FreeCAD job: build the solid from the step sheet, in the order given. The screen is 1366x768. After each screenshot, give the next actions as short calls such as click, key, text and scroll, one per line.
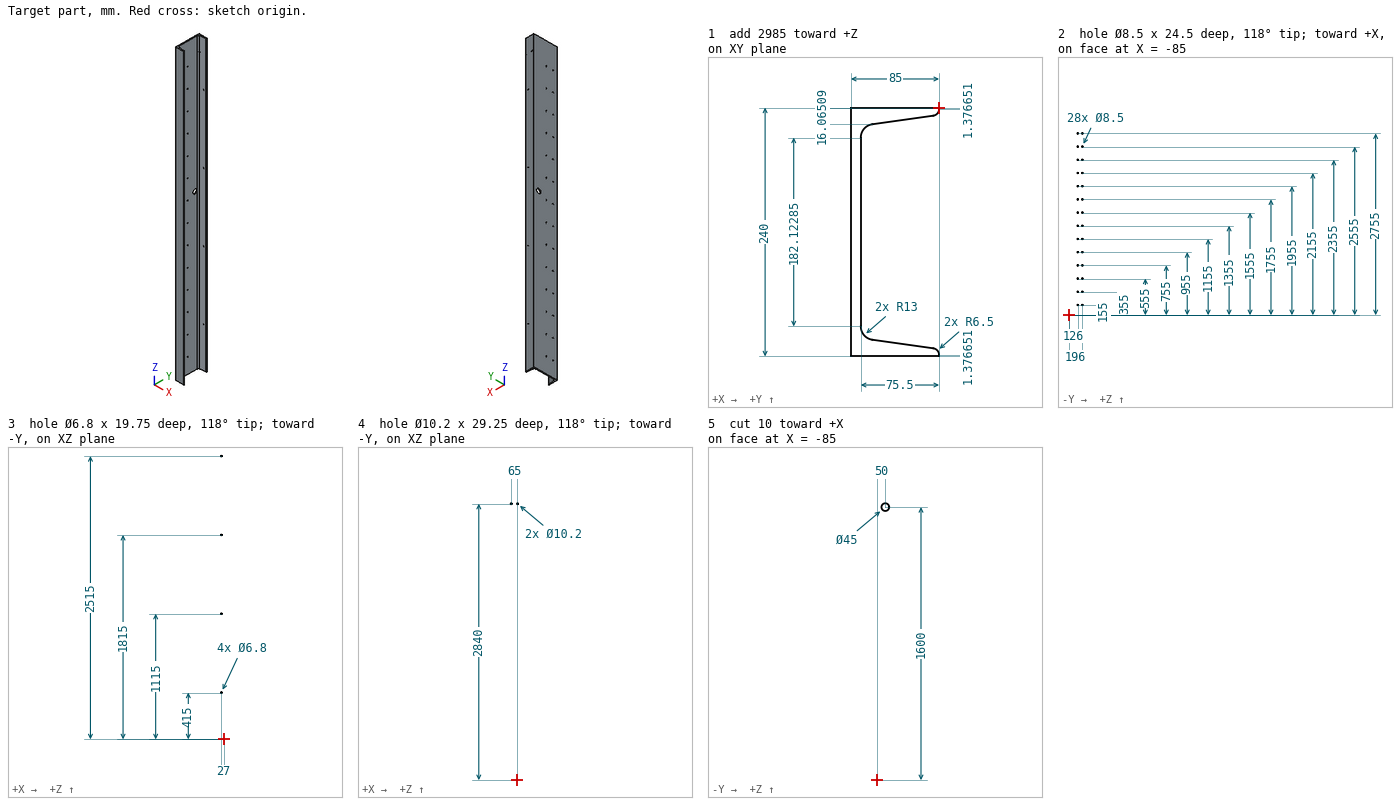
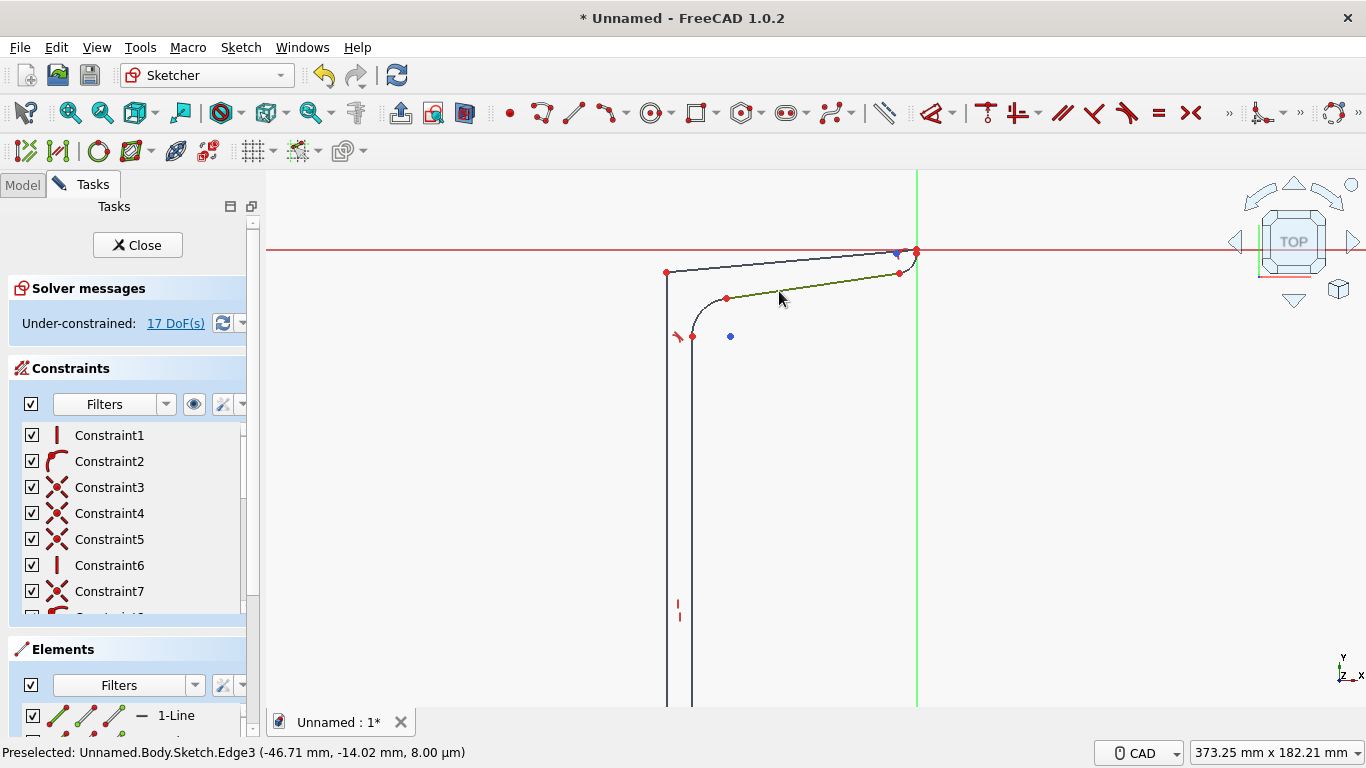
click(711, 304)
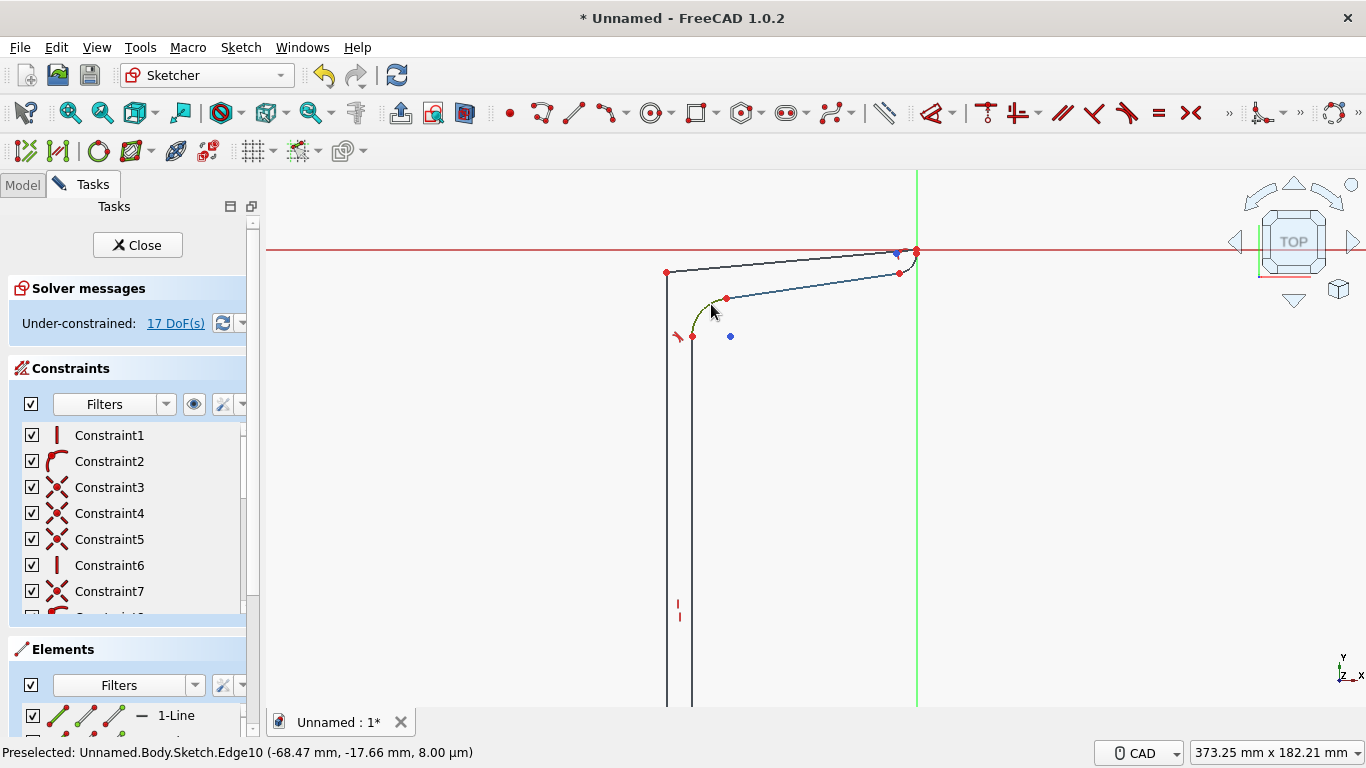
click(1128, 114)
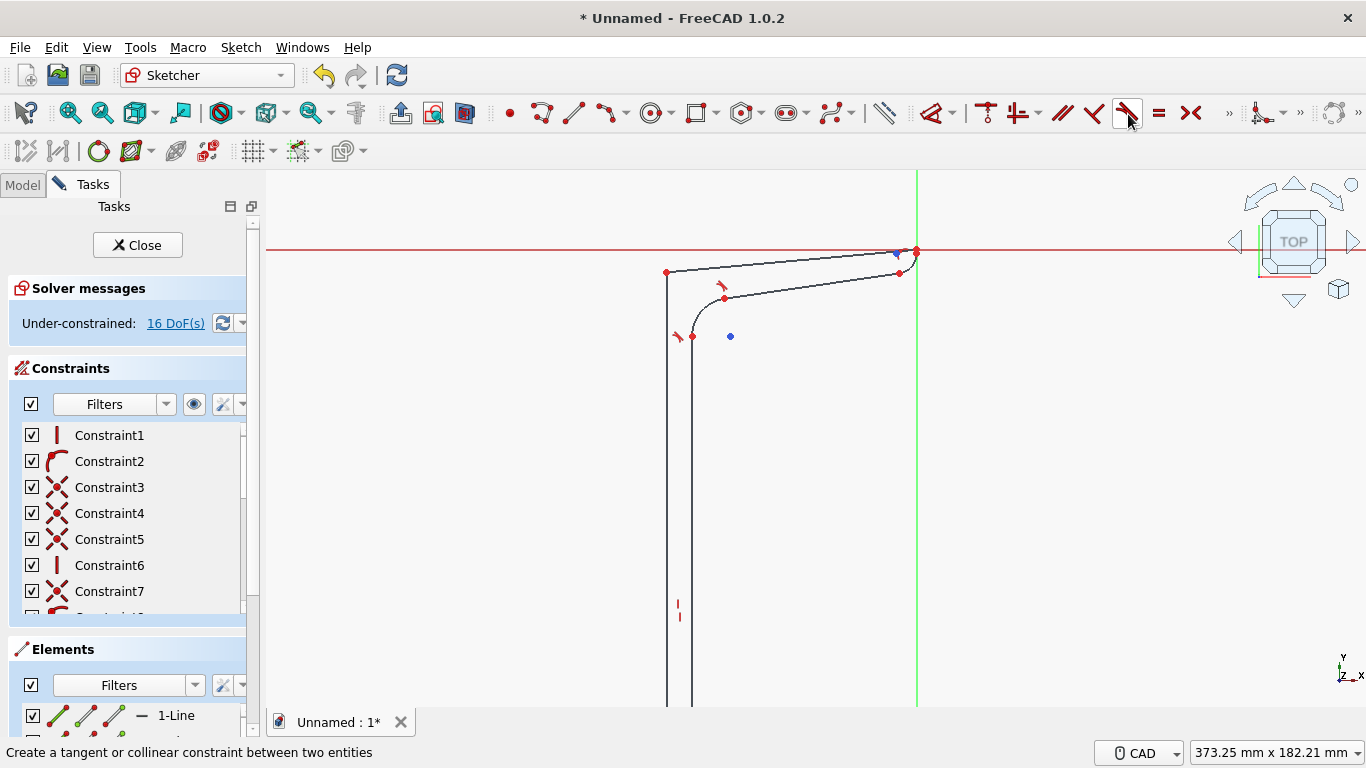
click(777, 291)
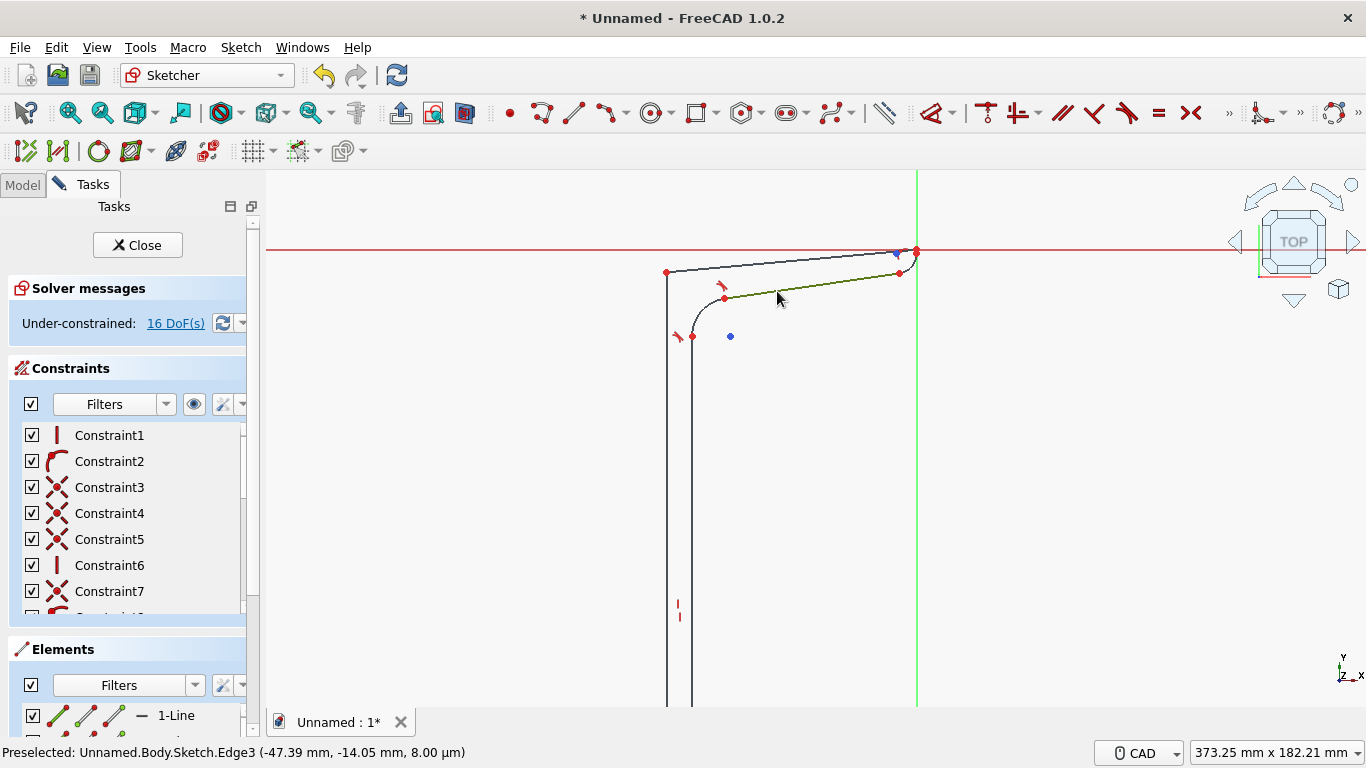
scroll(915, 262, up, 3)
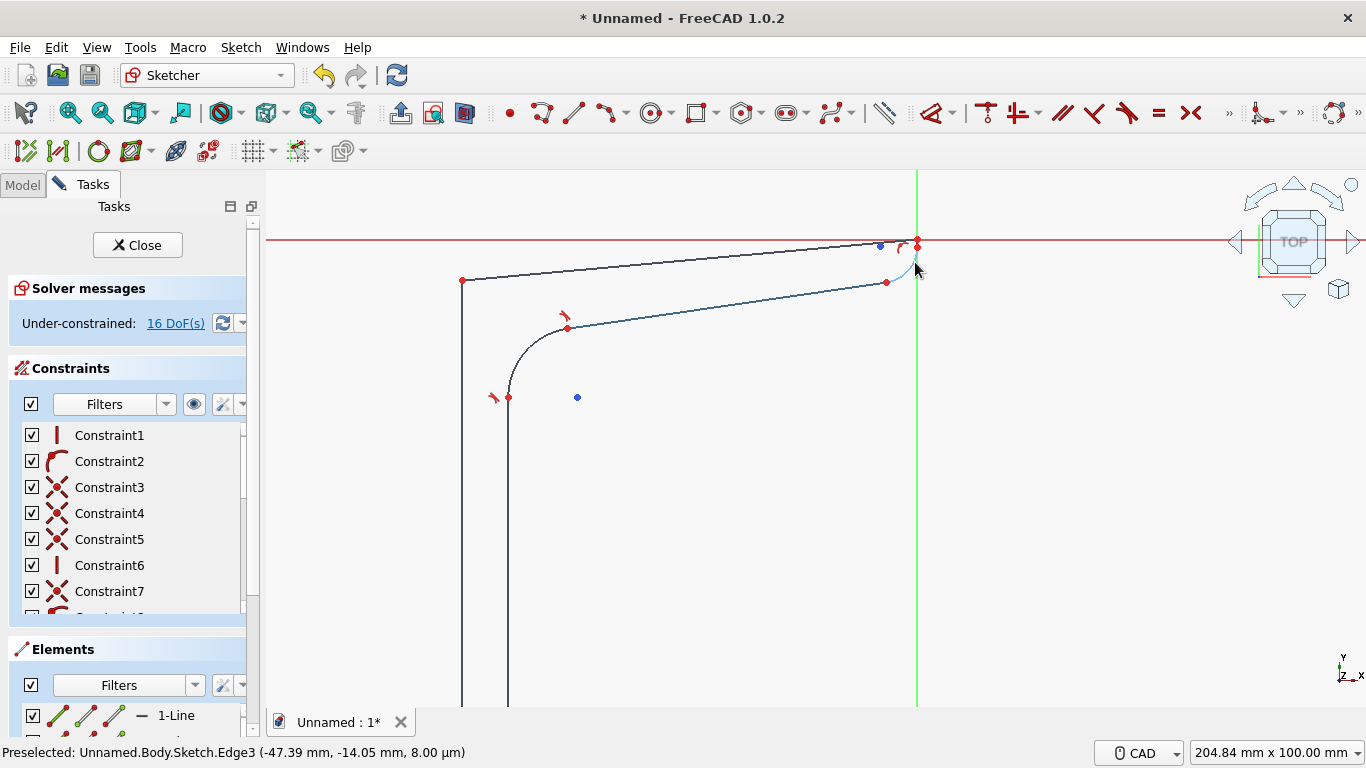
click(914, 262)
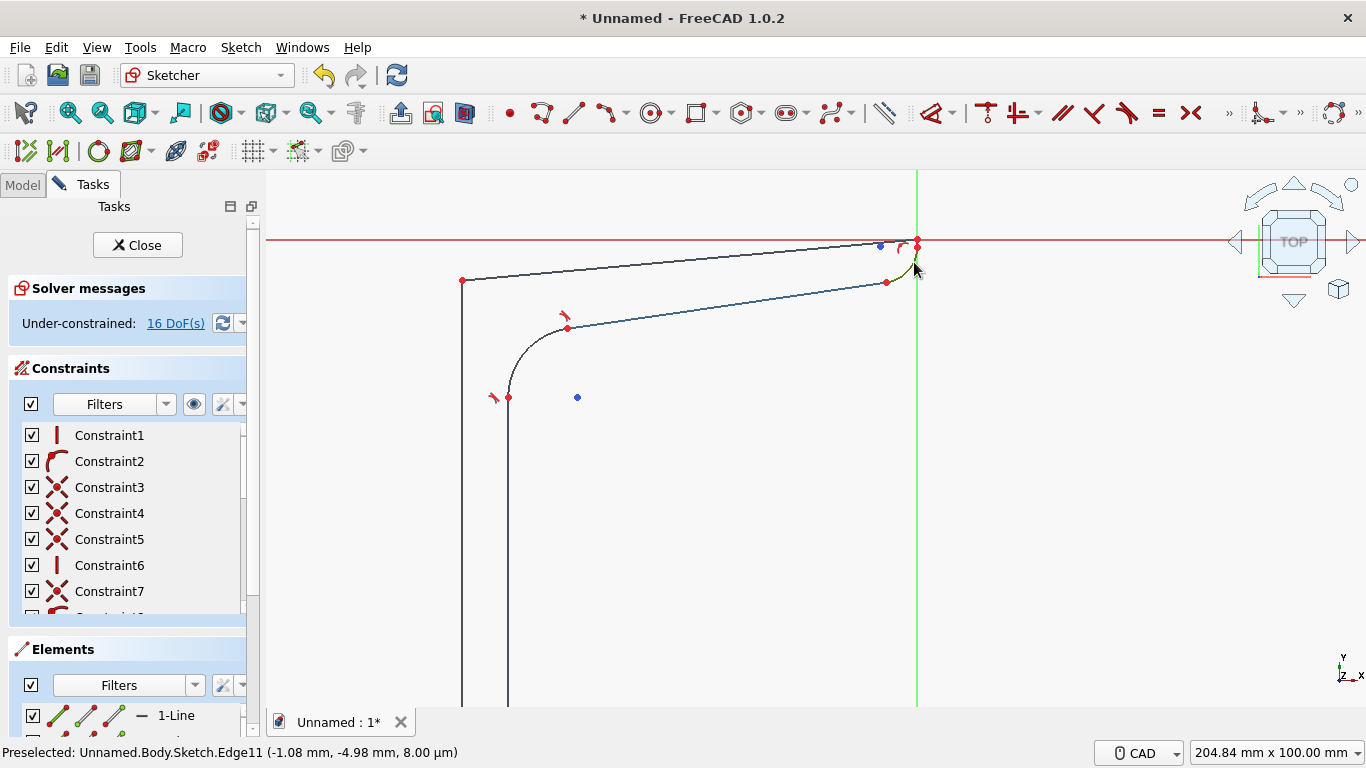
click(1128, 114)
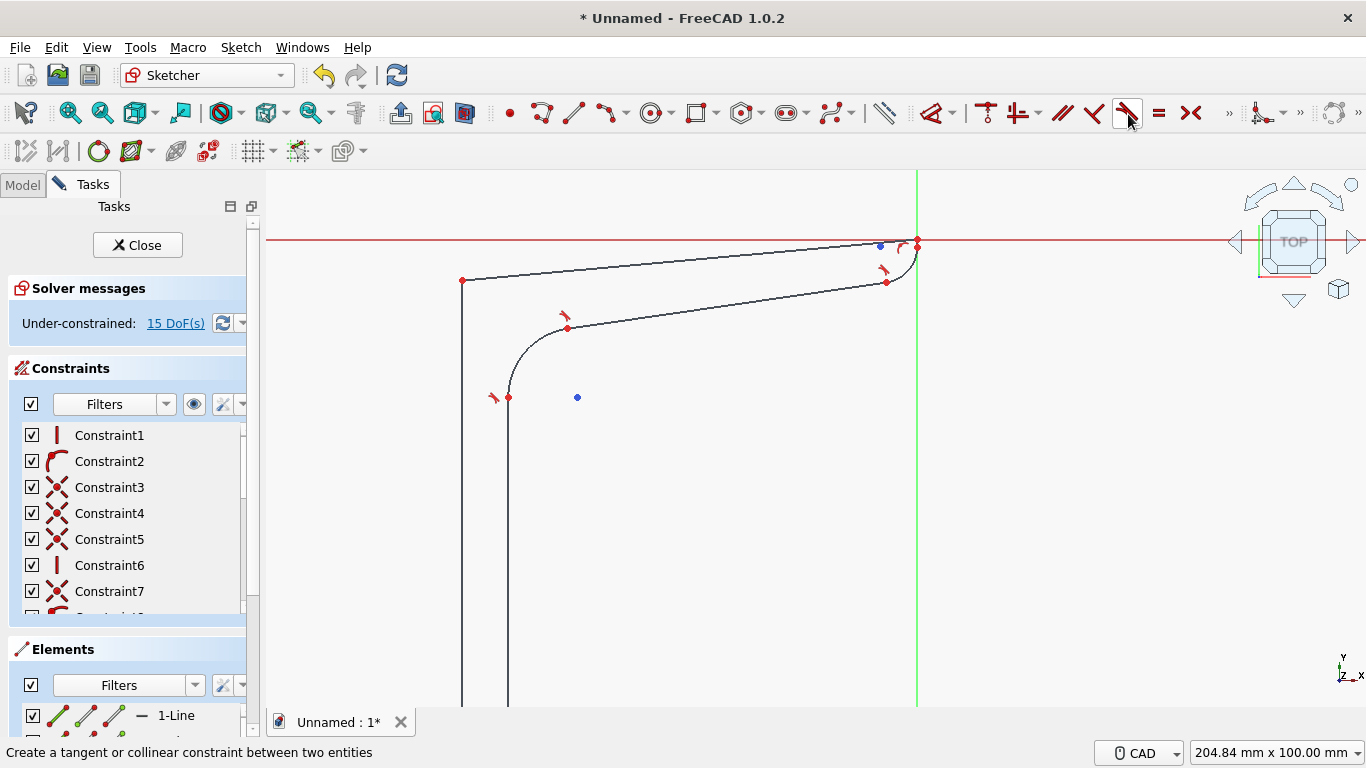
scroll(917, 243, up, 7)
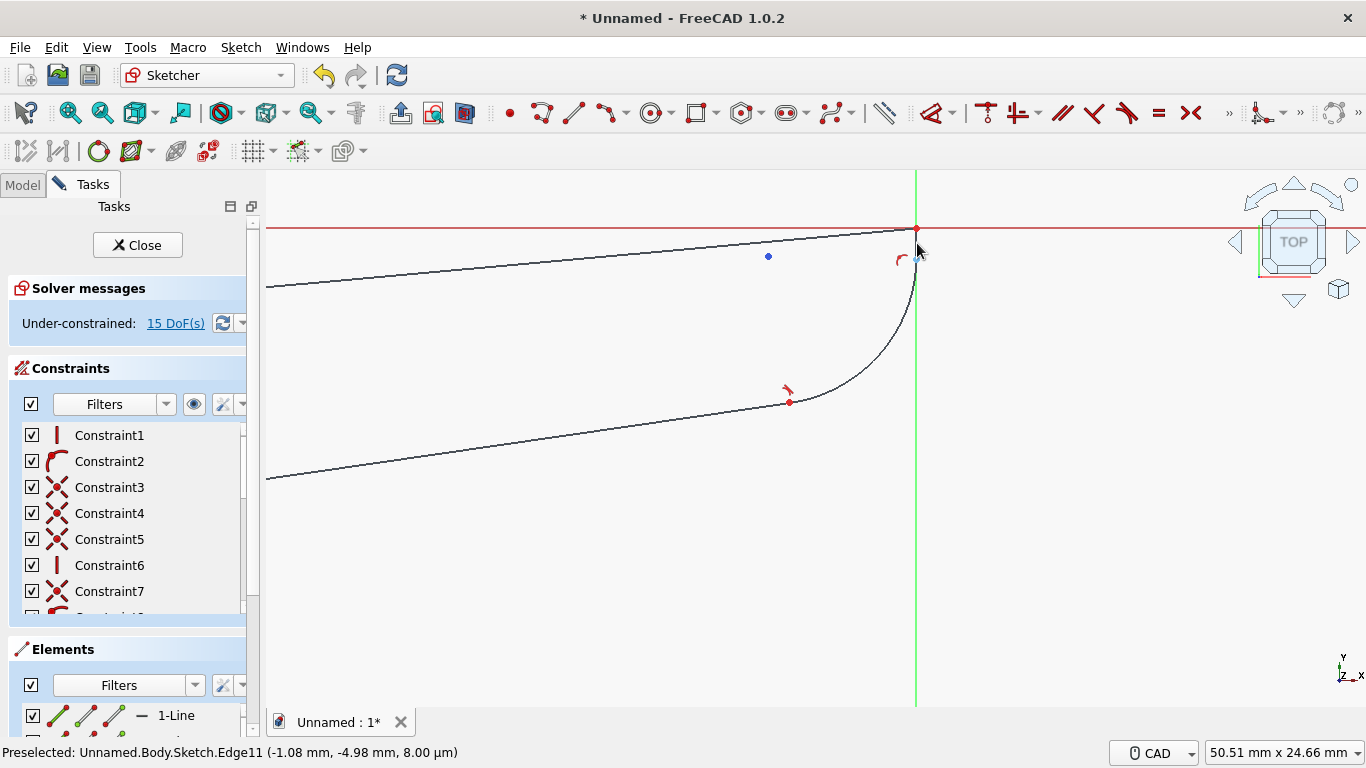
click(916, 244)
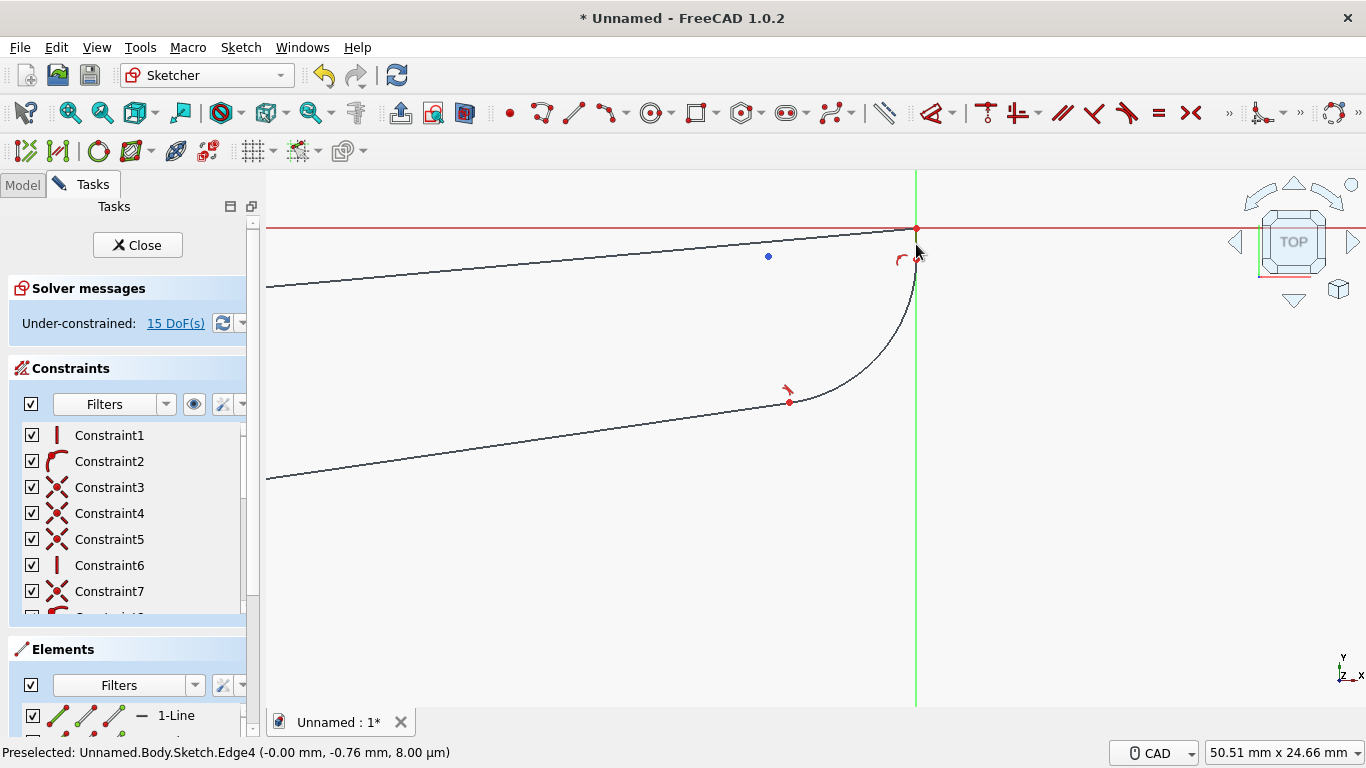
scroll(796, 283, down, 14)